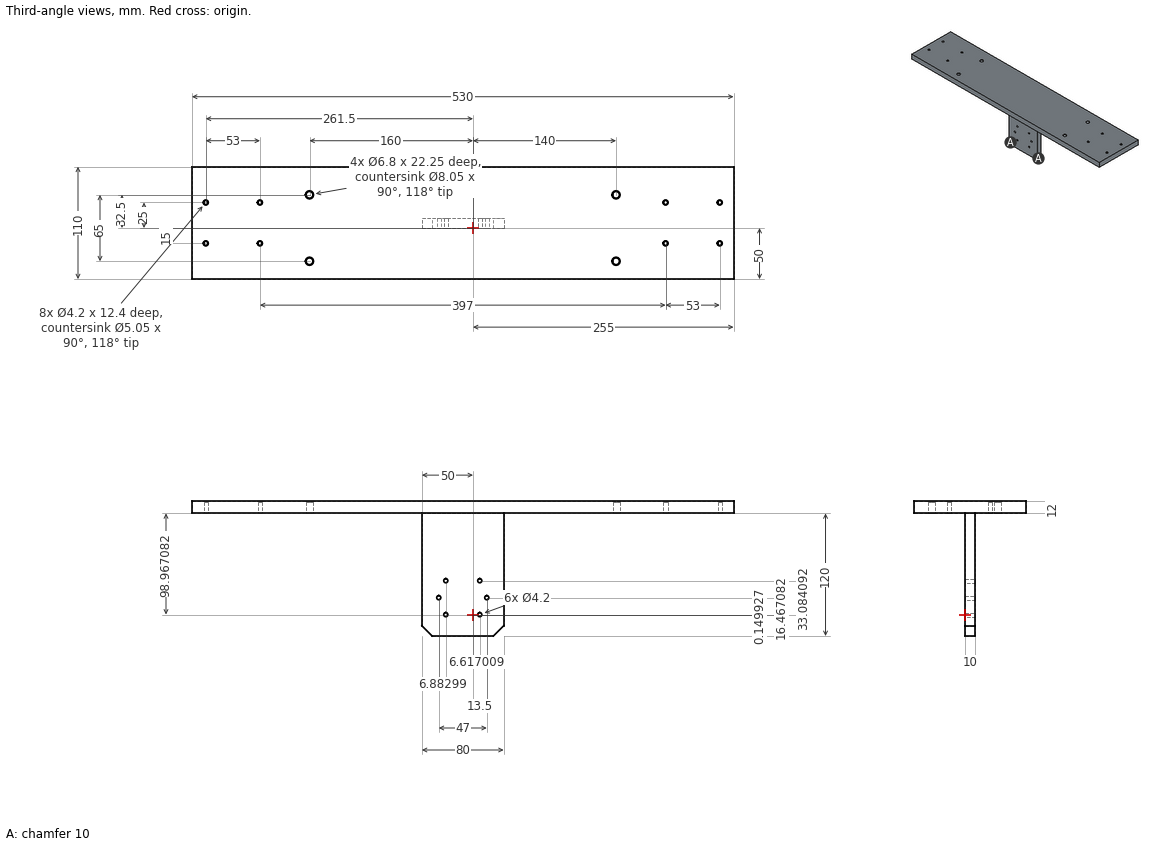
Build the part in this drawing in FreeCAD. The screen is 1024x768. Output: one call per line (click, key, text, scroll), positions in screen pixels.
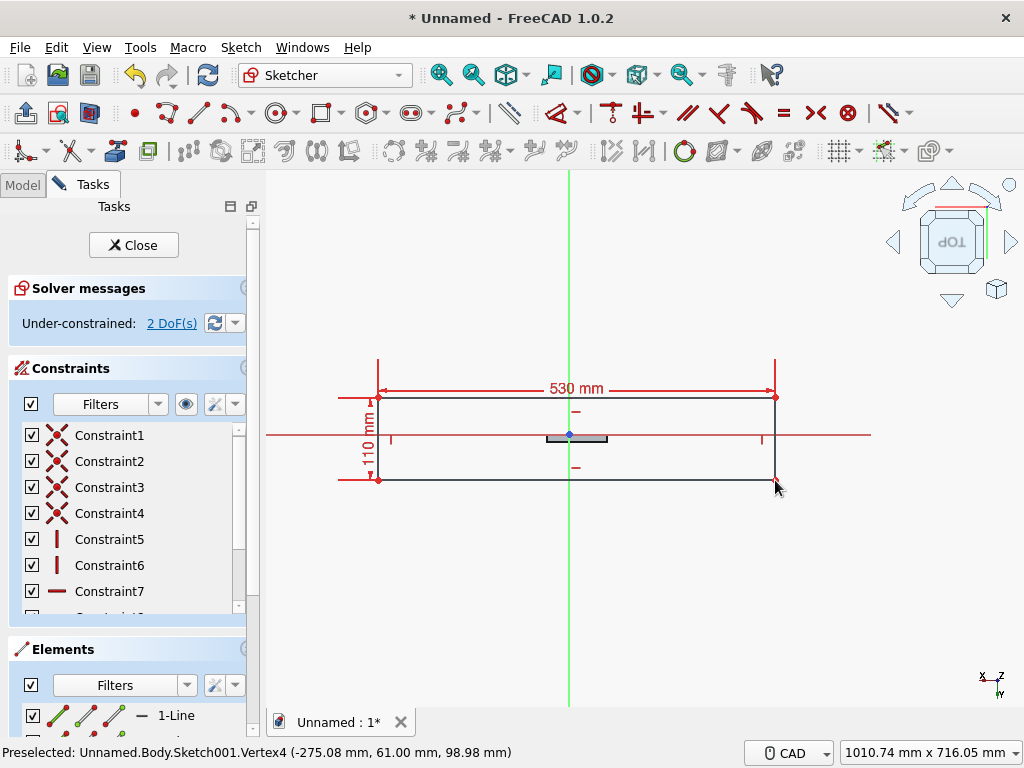
click(378, 398)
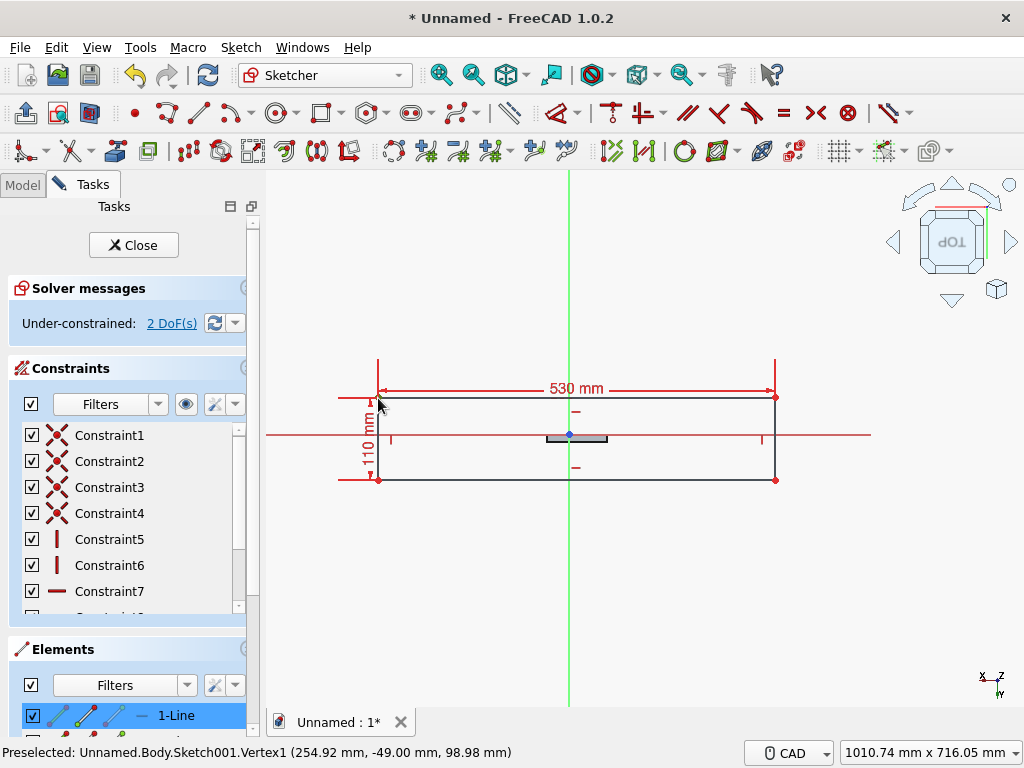
key(i)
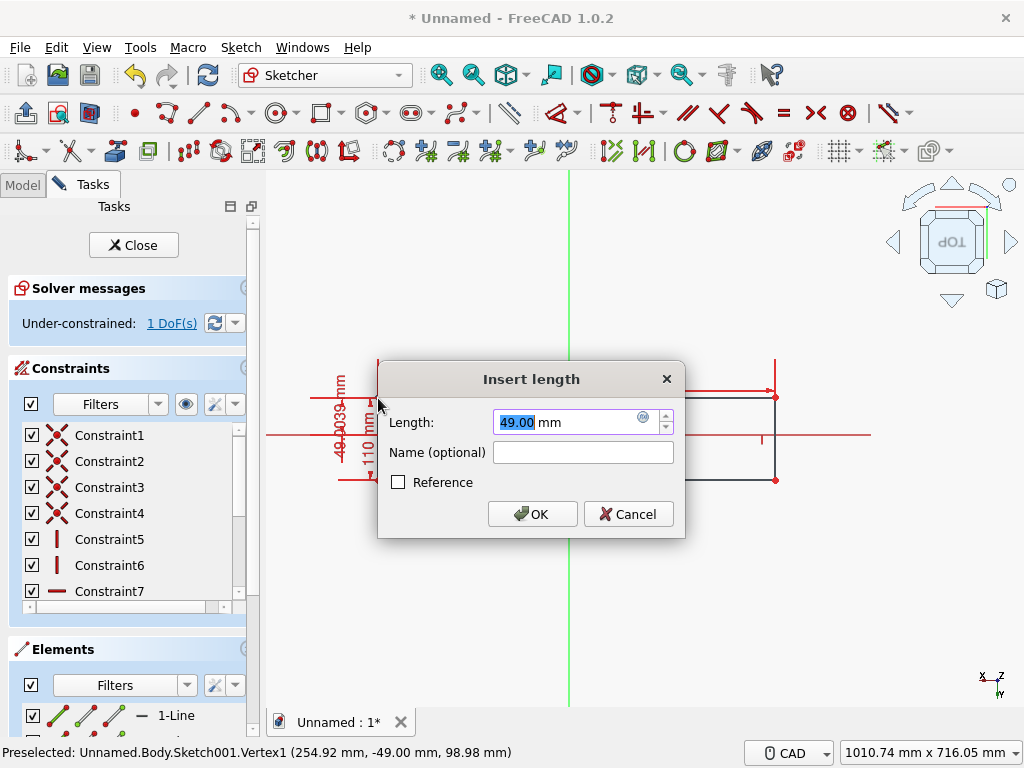
text(50)
key(Return)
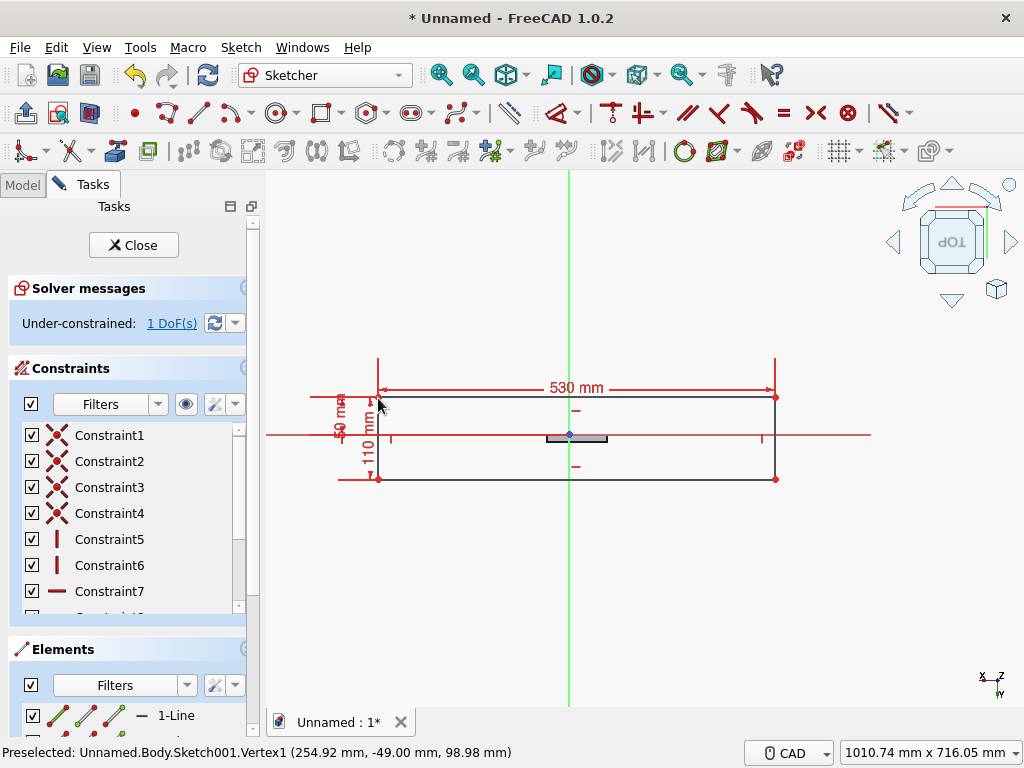
click(378, 397)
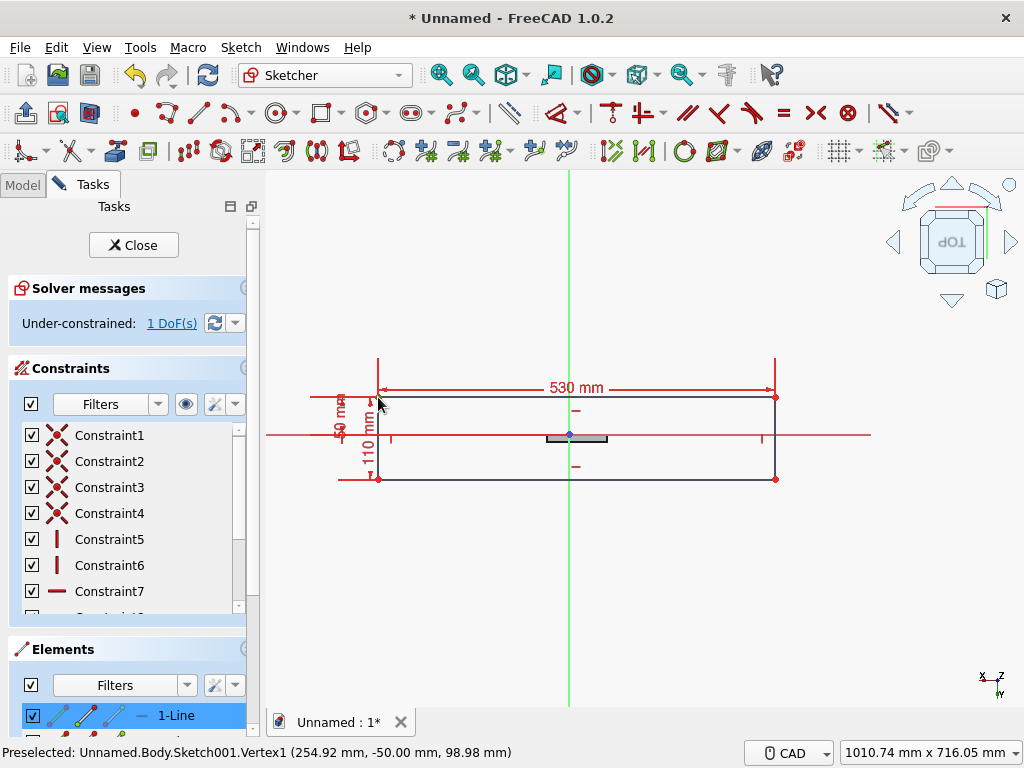
click(580, 114)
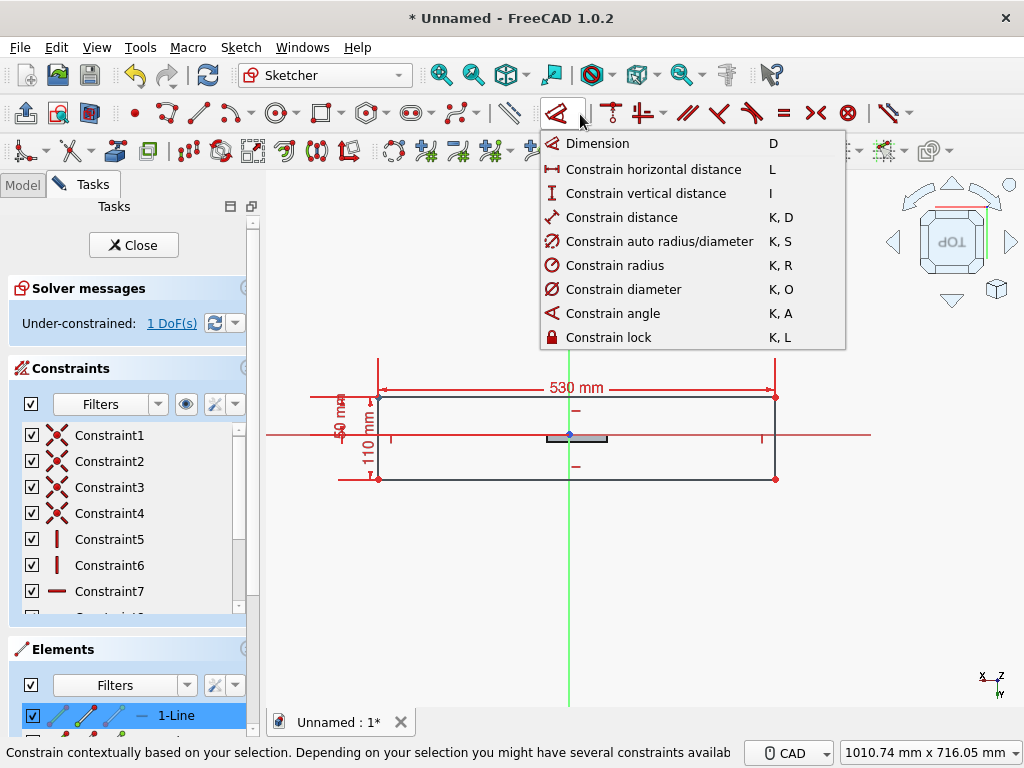
click(693, 169)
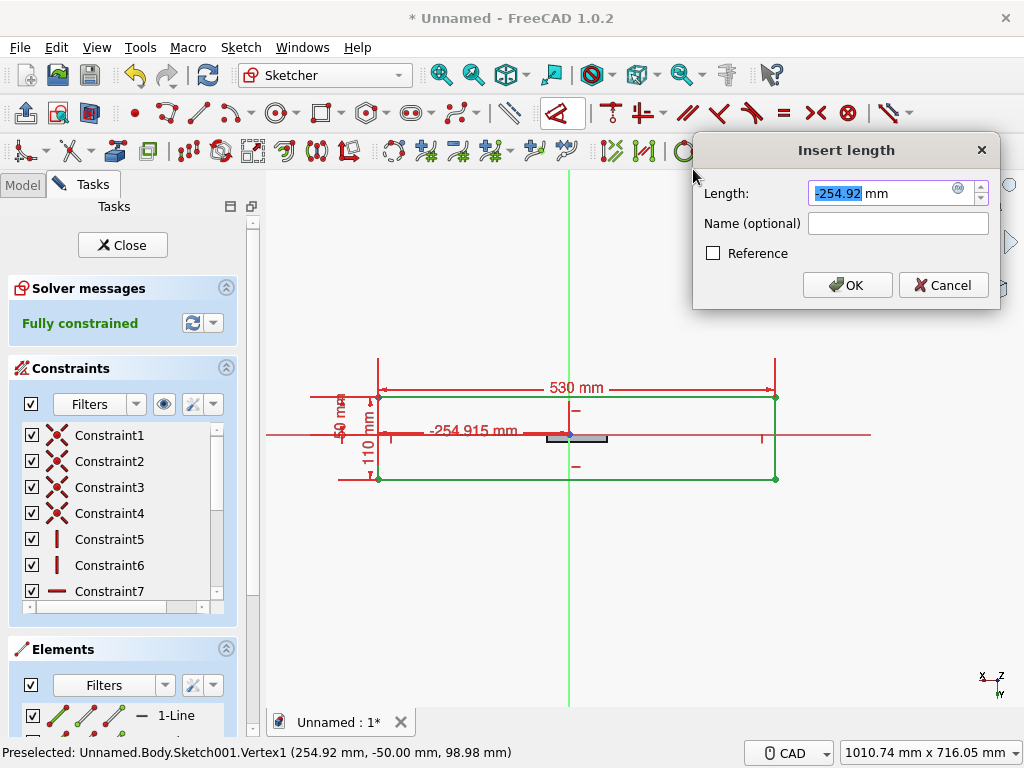
text(-255)
key(Return)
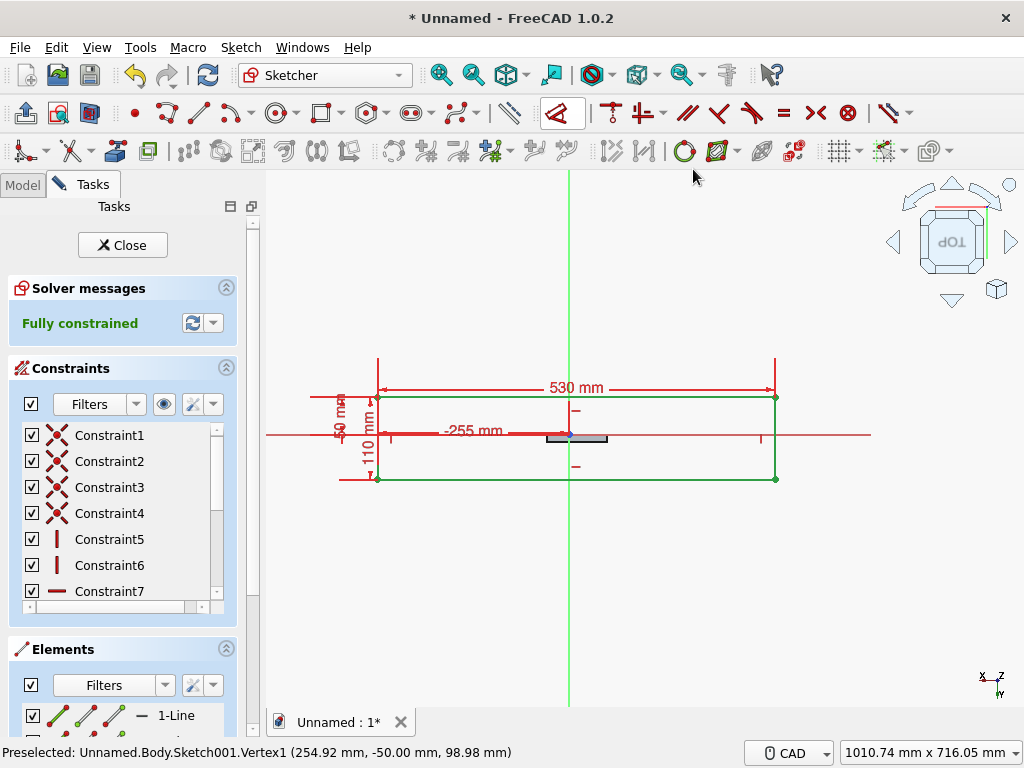
click(123, 245)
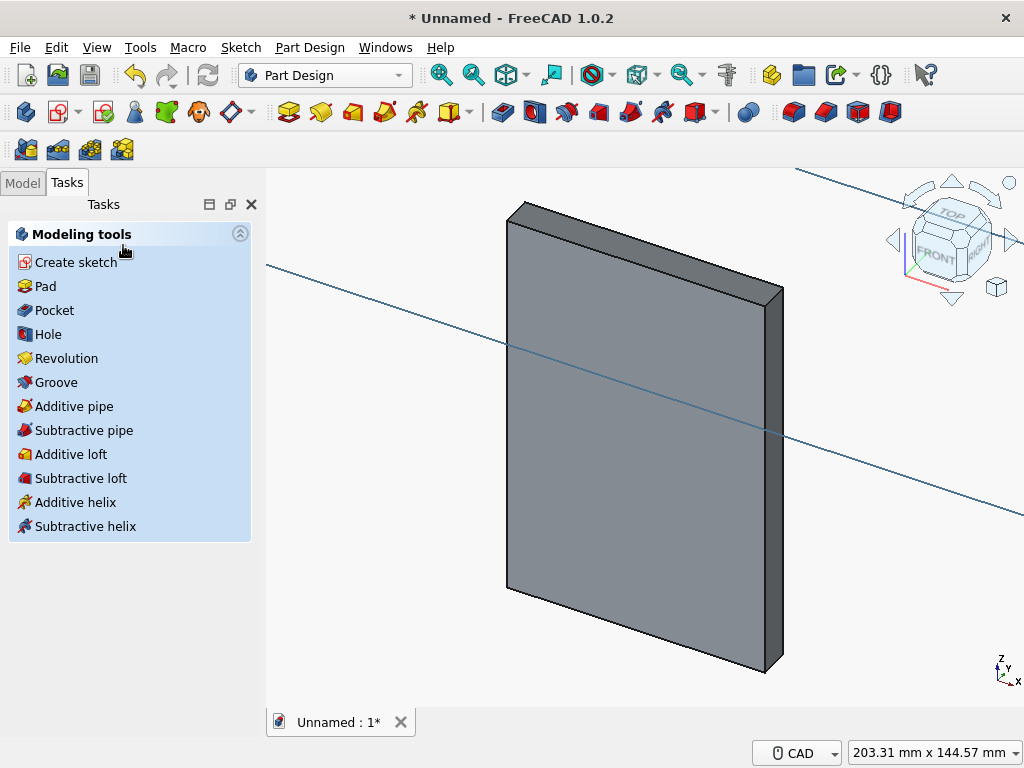
click(290, 112)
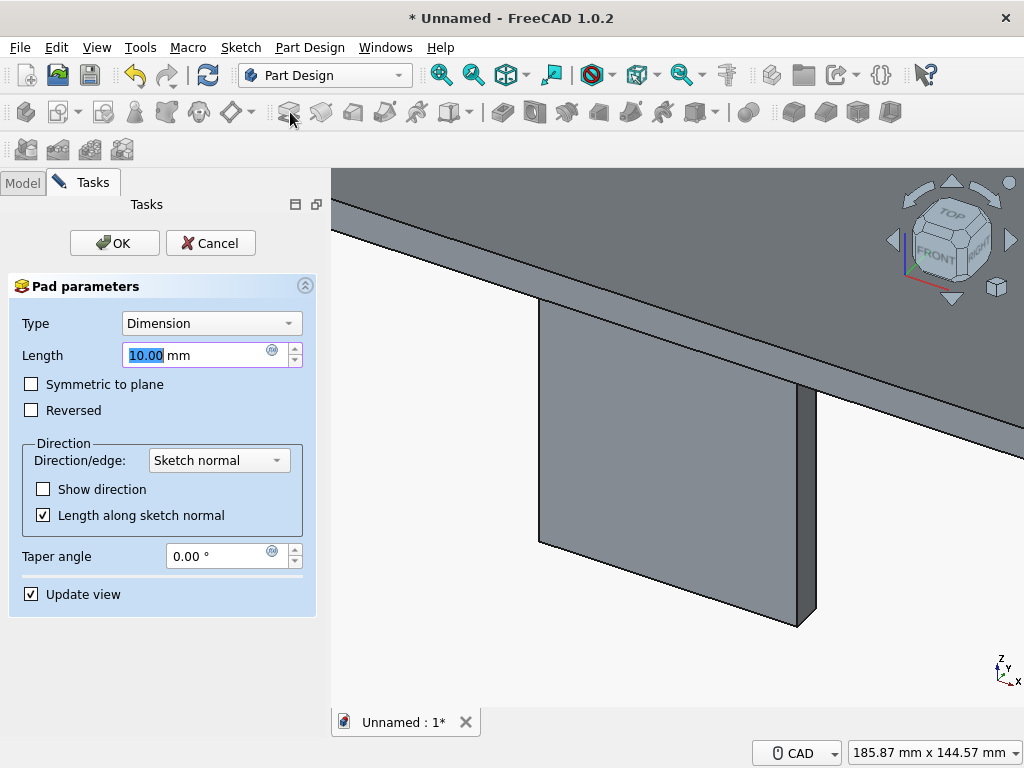
text(12)
key(Tab)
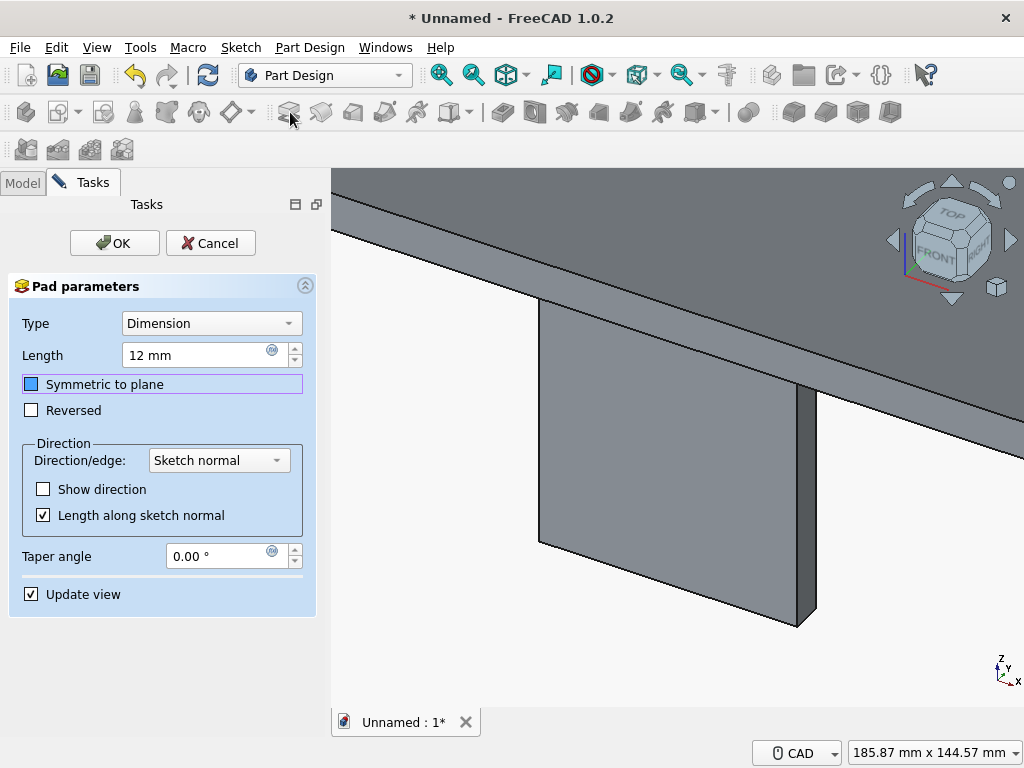
click(115, 243)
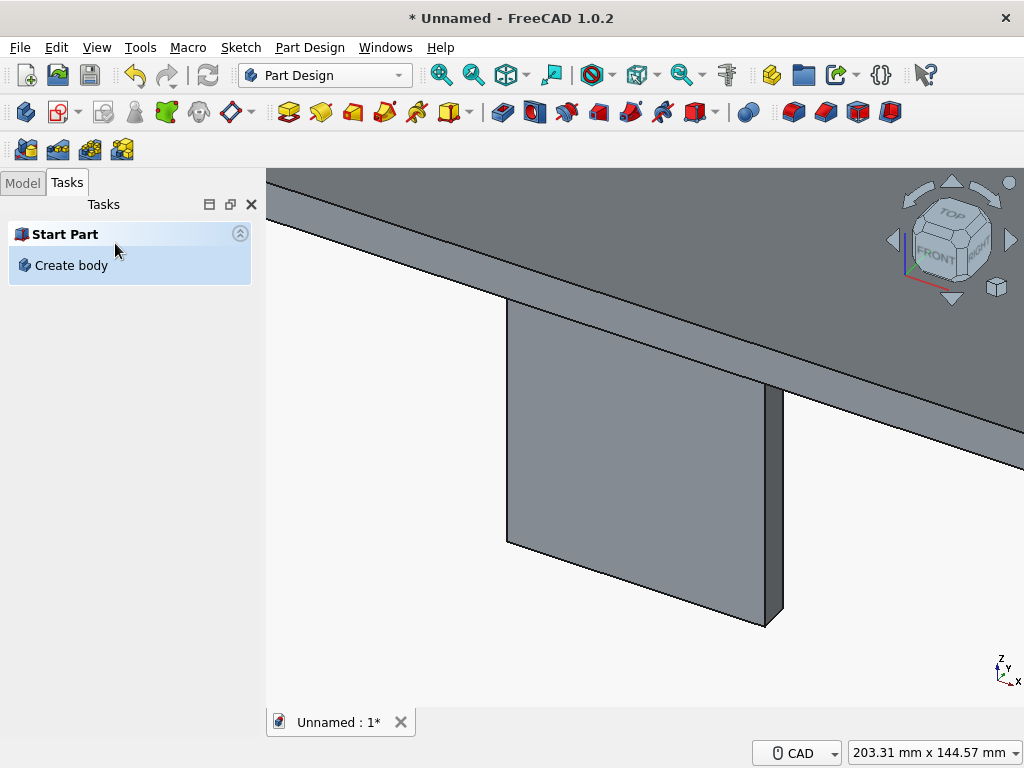
key(v)
key(f)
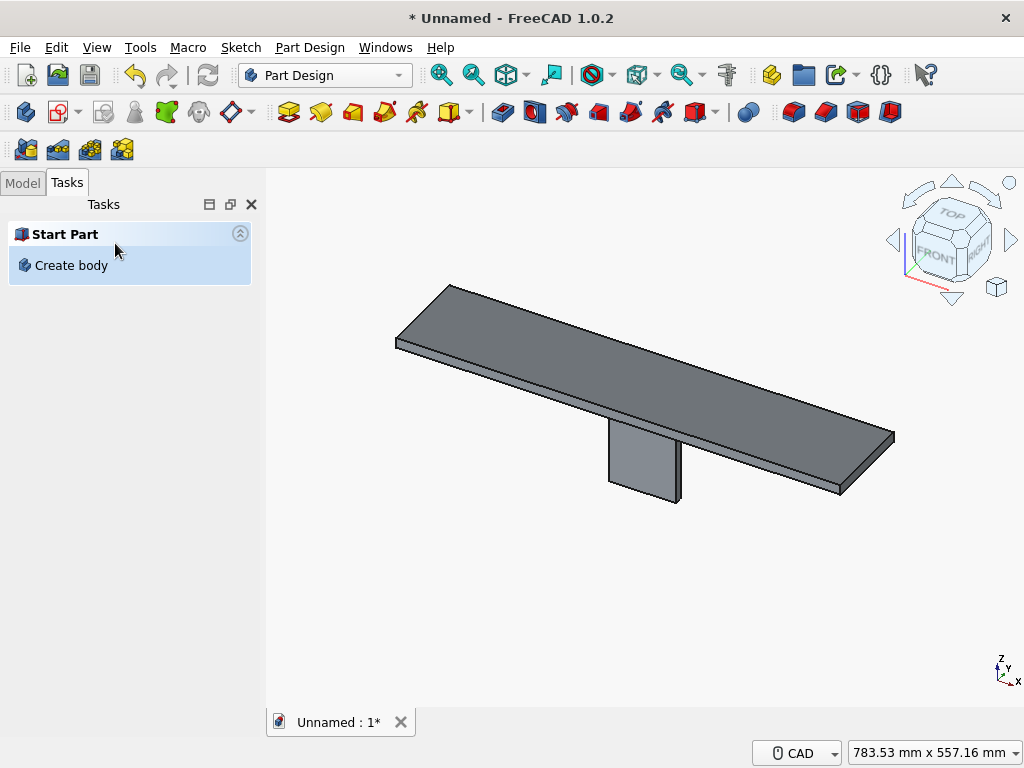
scroll(611, 478, up, 8)